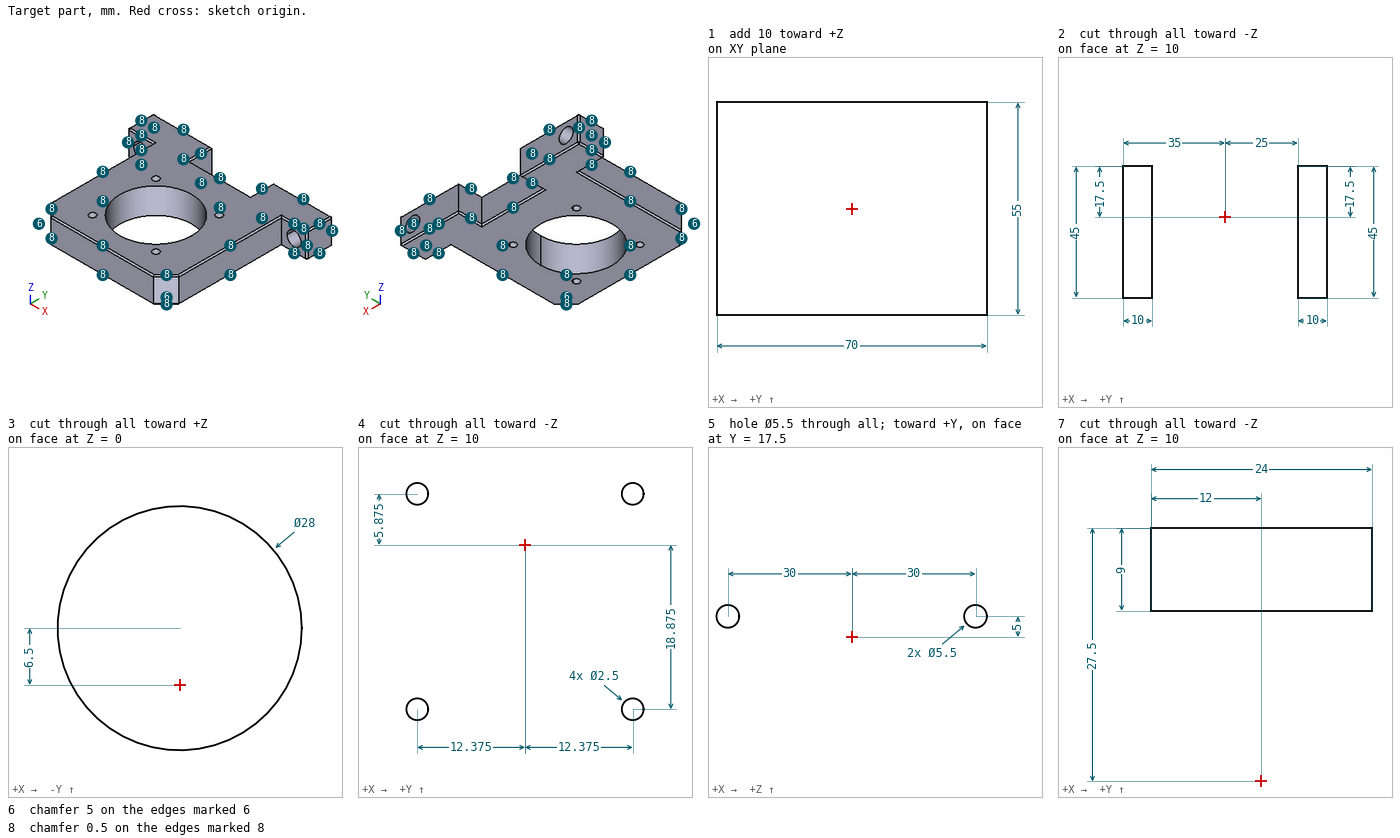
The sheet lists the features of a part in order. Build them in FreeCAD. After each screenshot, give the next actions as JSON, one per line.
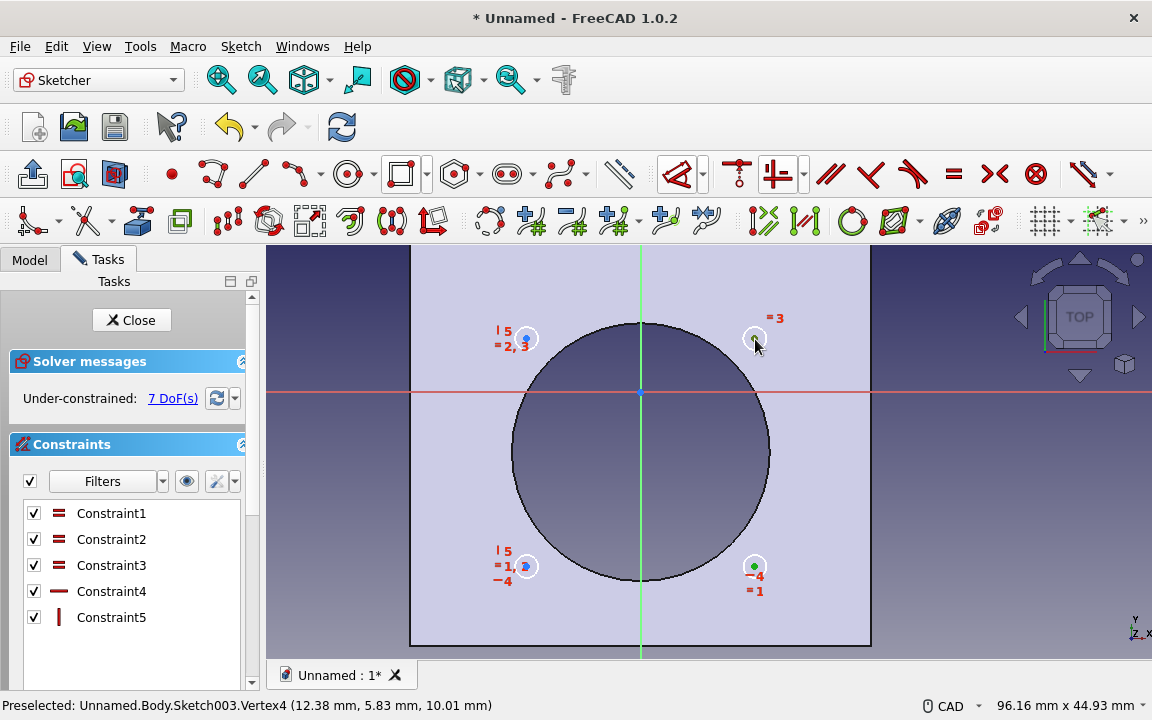
{"action": "left_click", "coordinate": [804, 174]}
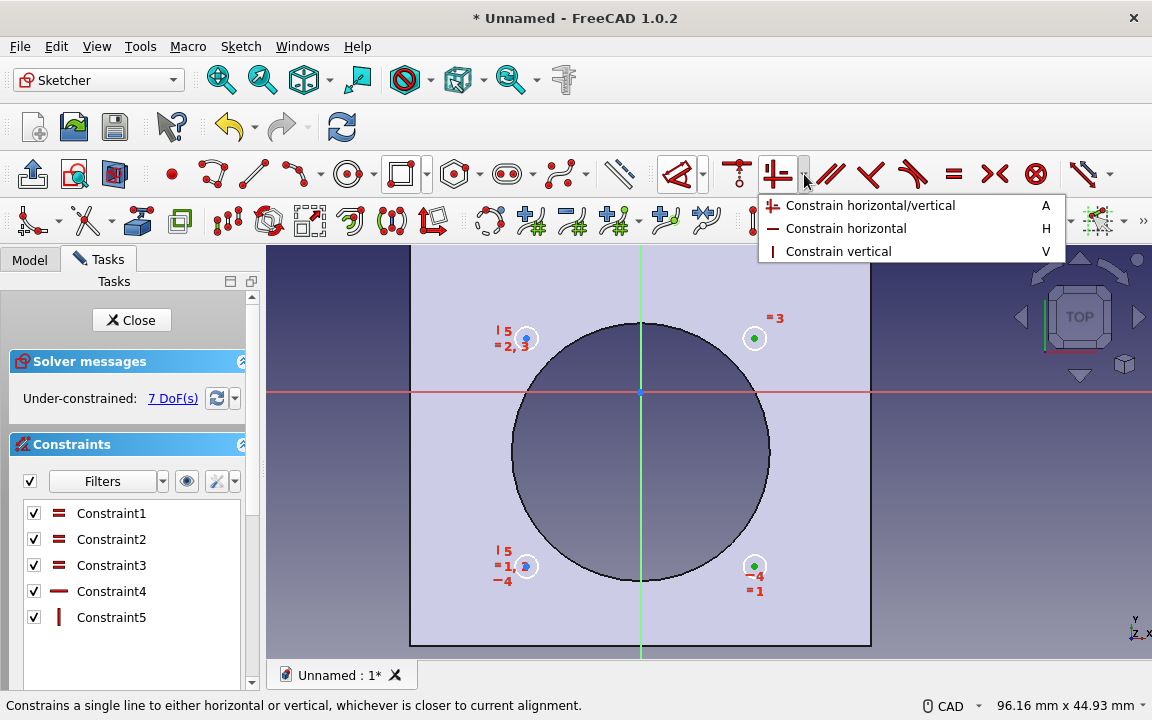
{"action": "left_click", "coordinate": [912, 252]}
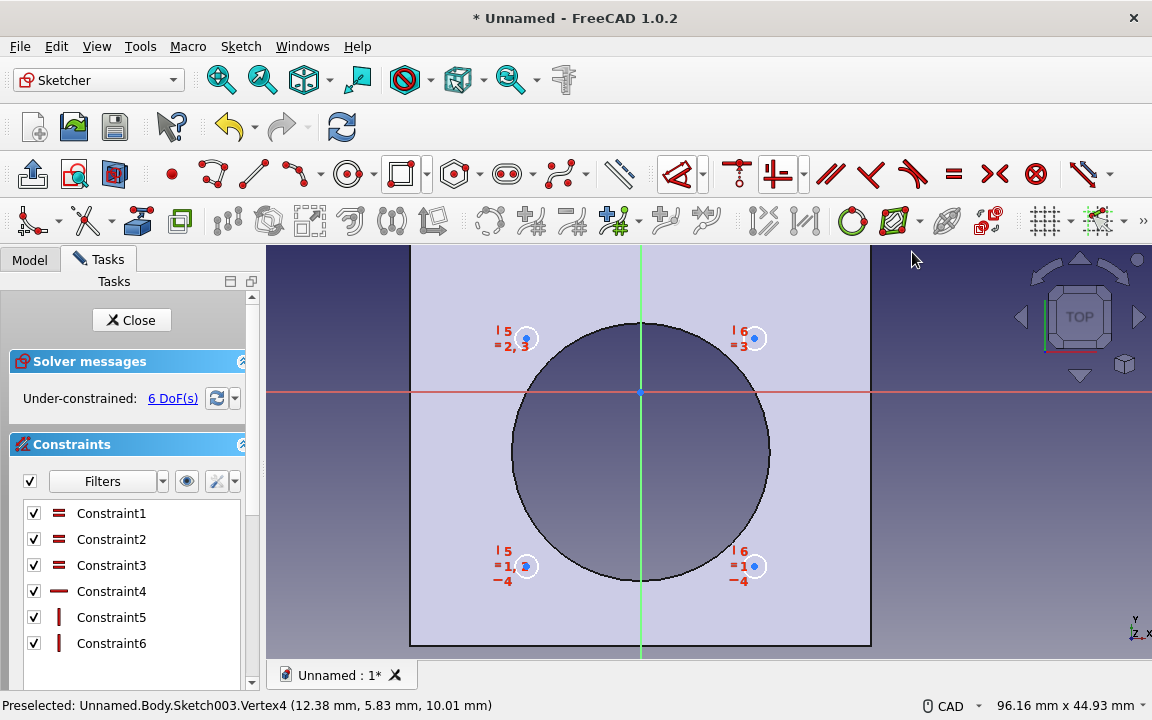
{"action": "left_click", "coordinate": [529, 341]}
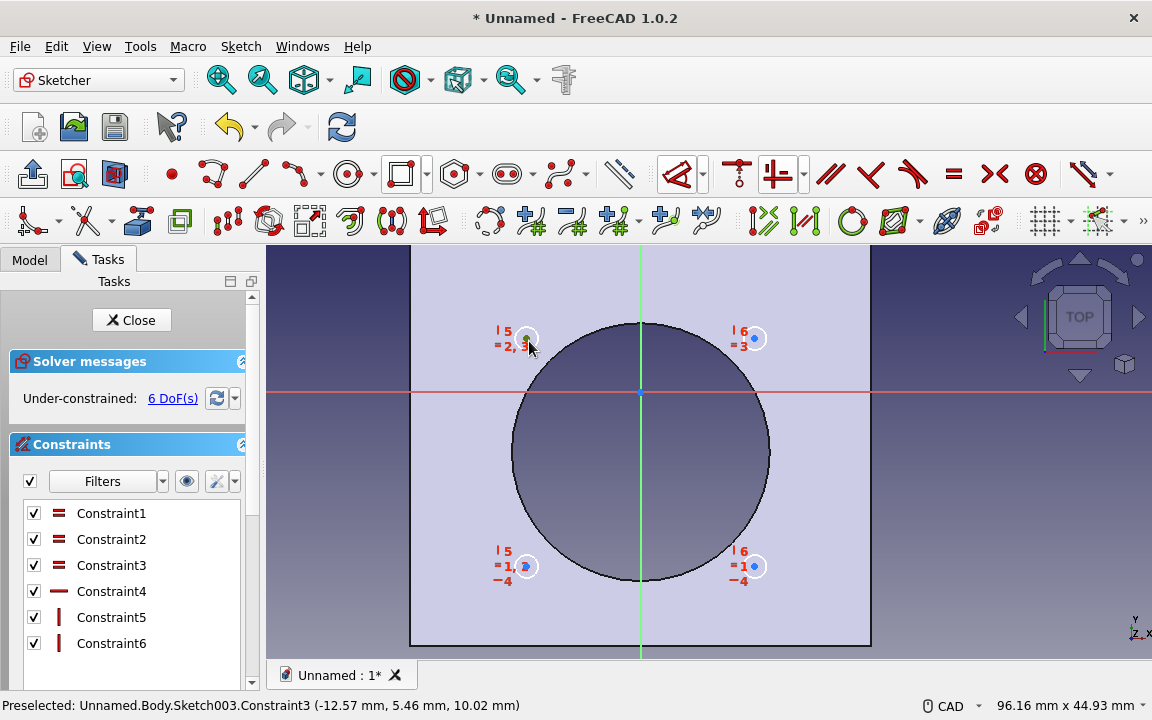
{"action": "left_click", "coordinate": [755, 339]}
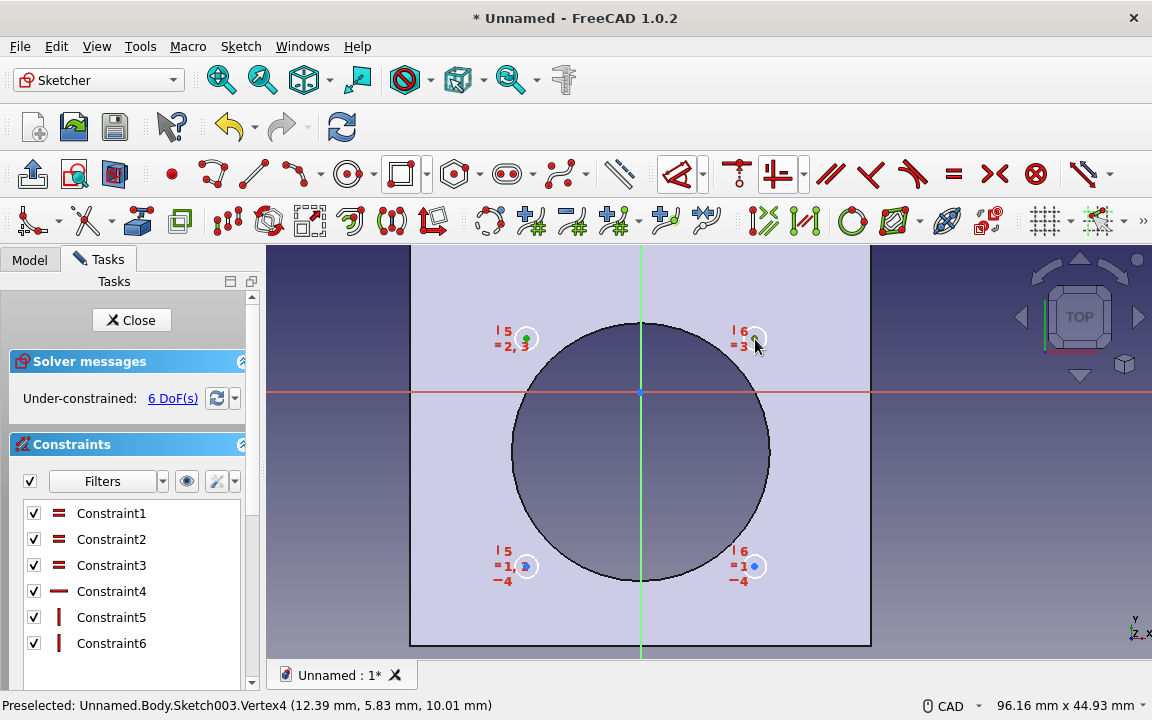
{"action": "left_click", "coordinate": [804, 174]}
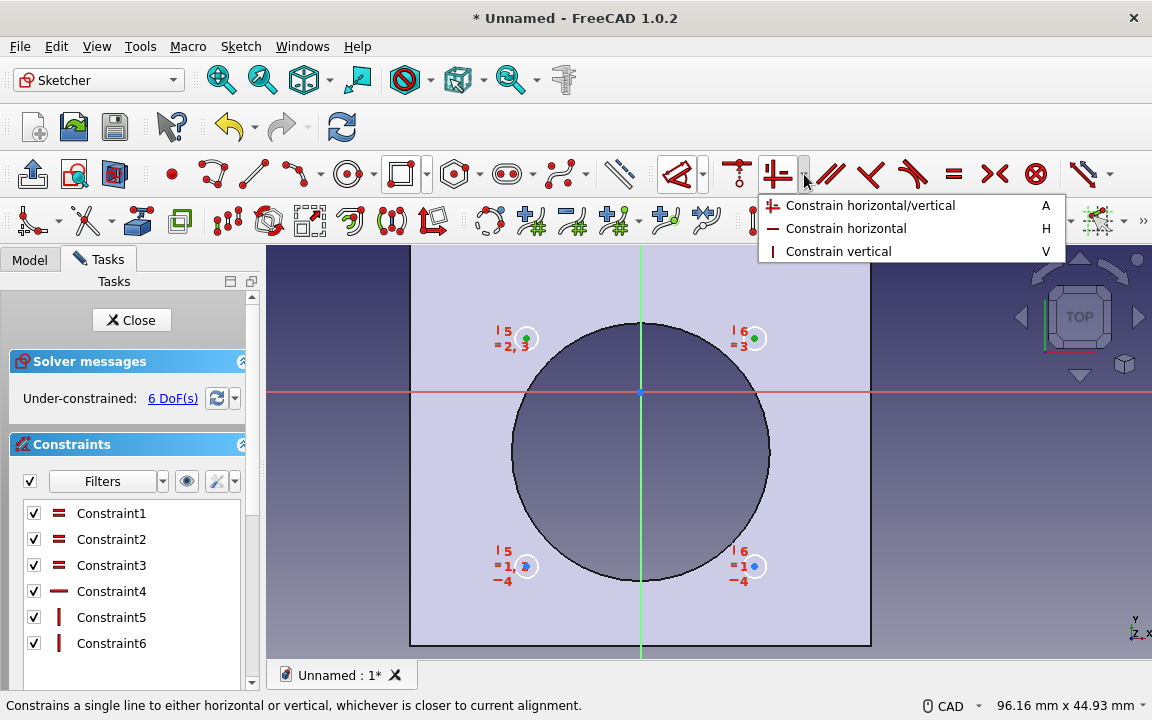
{"action": "left_click", "coordinate": [912, 228]}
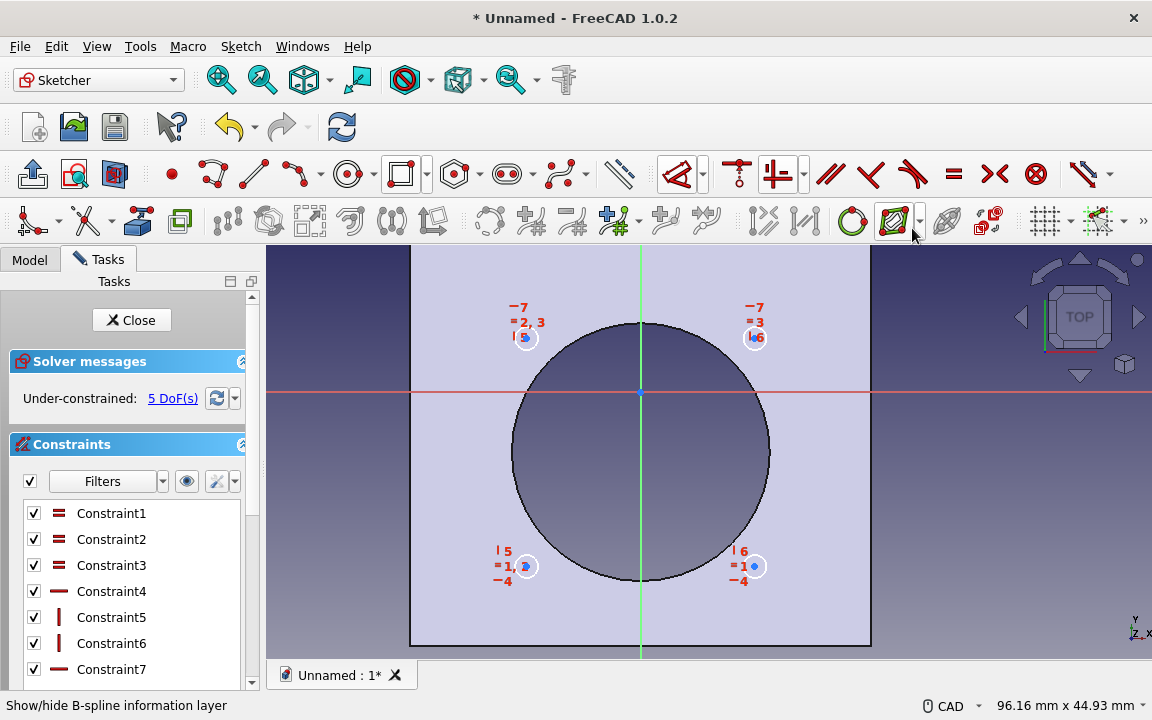
{"action": "scroll", "coordinate": [763, 558], "scroll_direction": "up", "scroll_amount": 3}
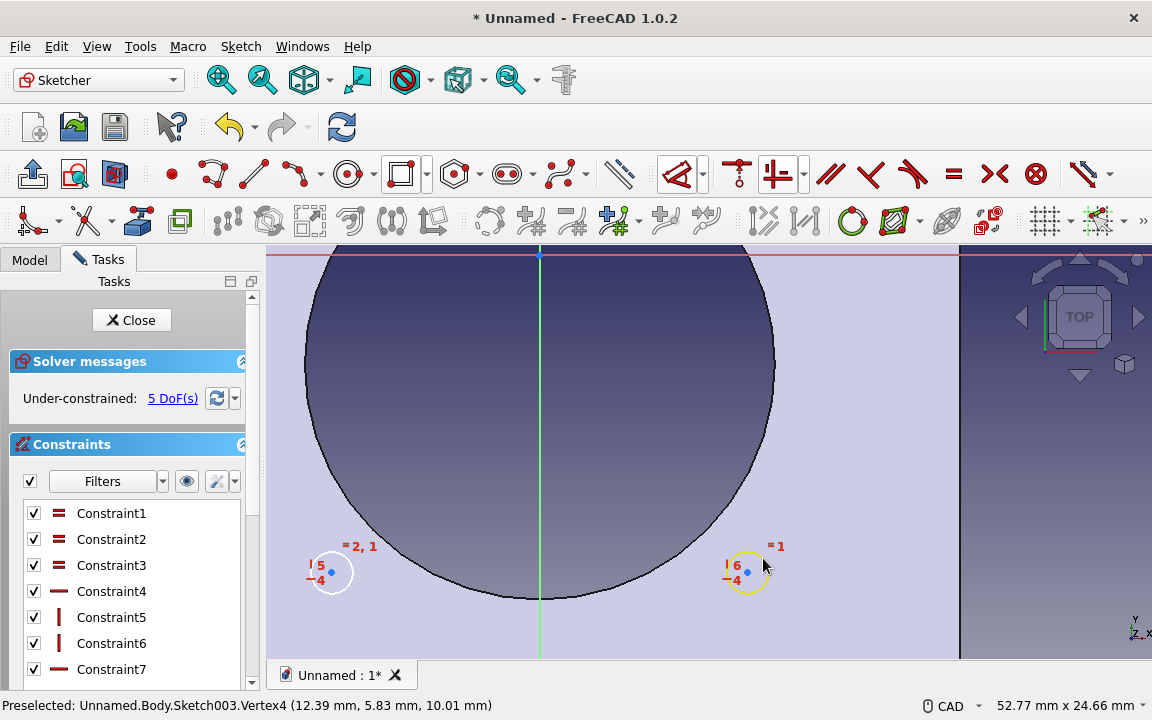
{"action": "left_click", "coordinate": [763, 558]}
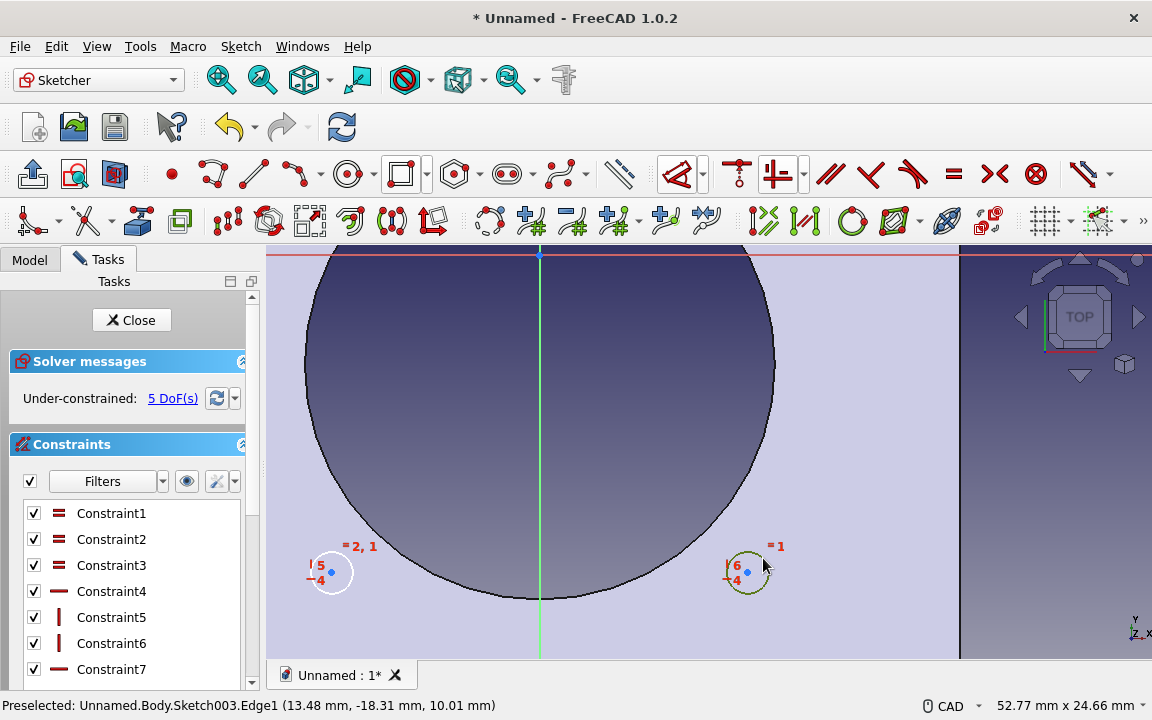
{"action": "key", "text": "k o"}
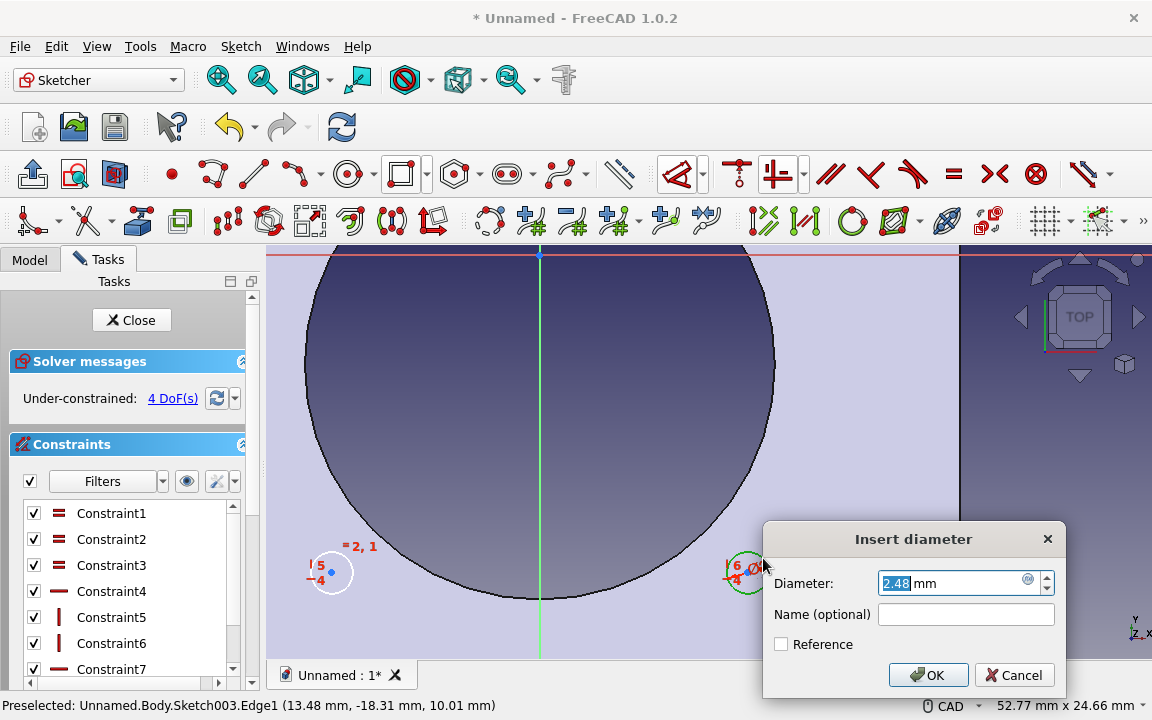
{"action": "type", "text": "2.5"}
{"action": "key", "text": "Return"}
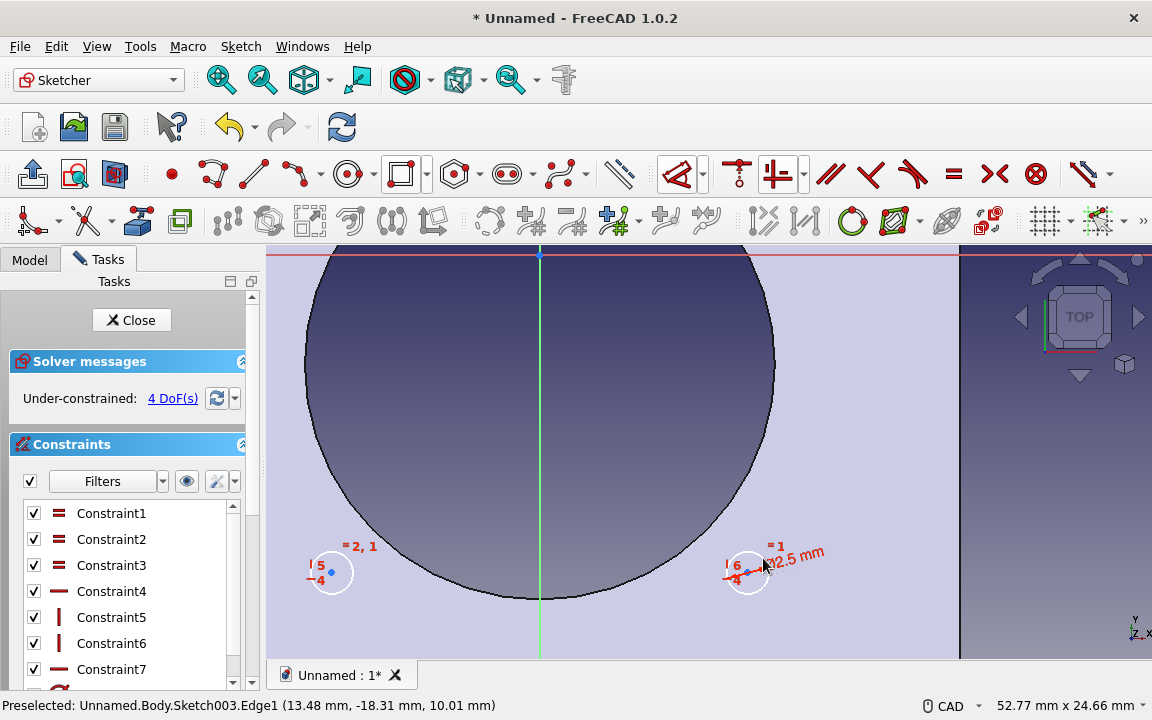
{"action": "scroll", "coordinate": [763, 558], "scroll_direction": "down", "scroll_amount": 3}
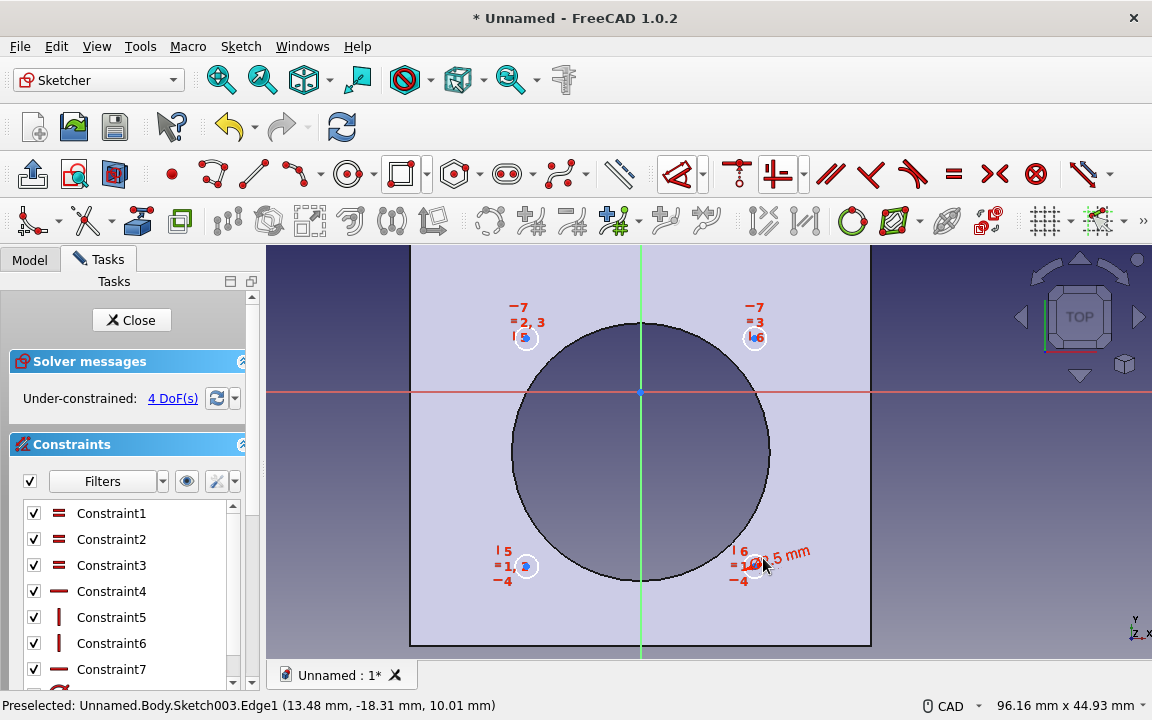
{"action": "left_click", "coordinate": [527, 339]}